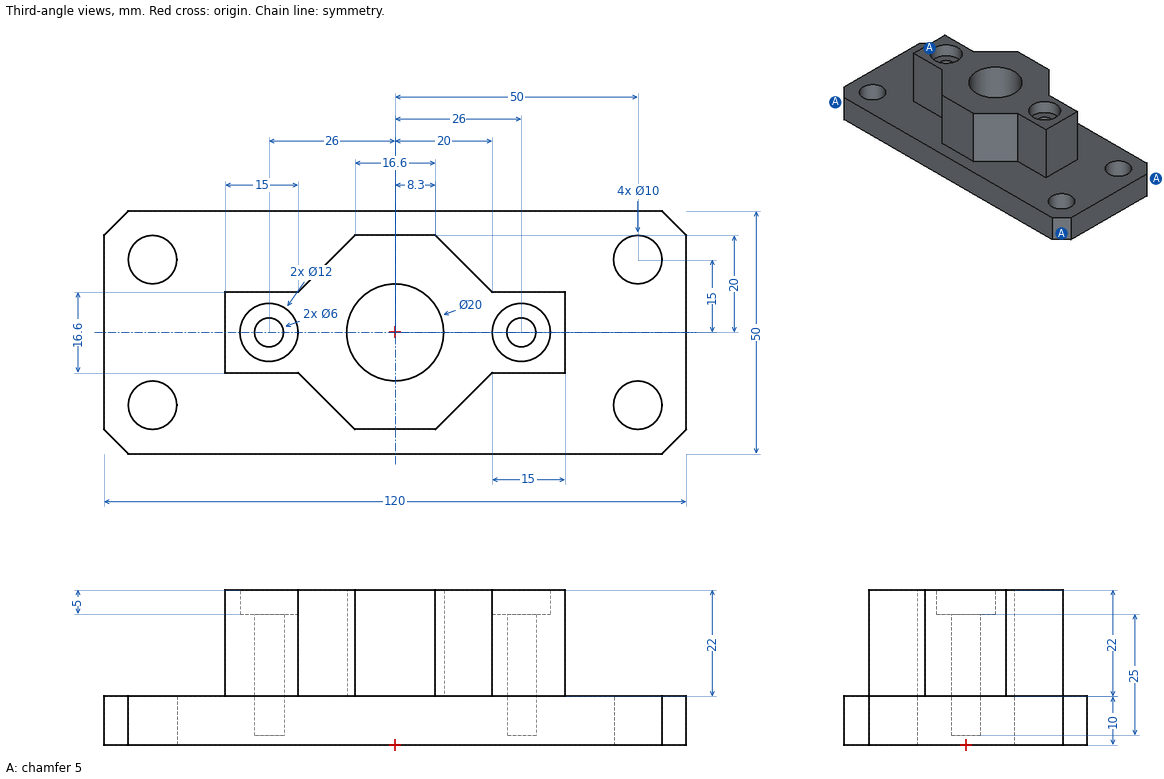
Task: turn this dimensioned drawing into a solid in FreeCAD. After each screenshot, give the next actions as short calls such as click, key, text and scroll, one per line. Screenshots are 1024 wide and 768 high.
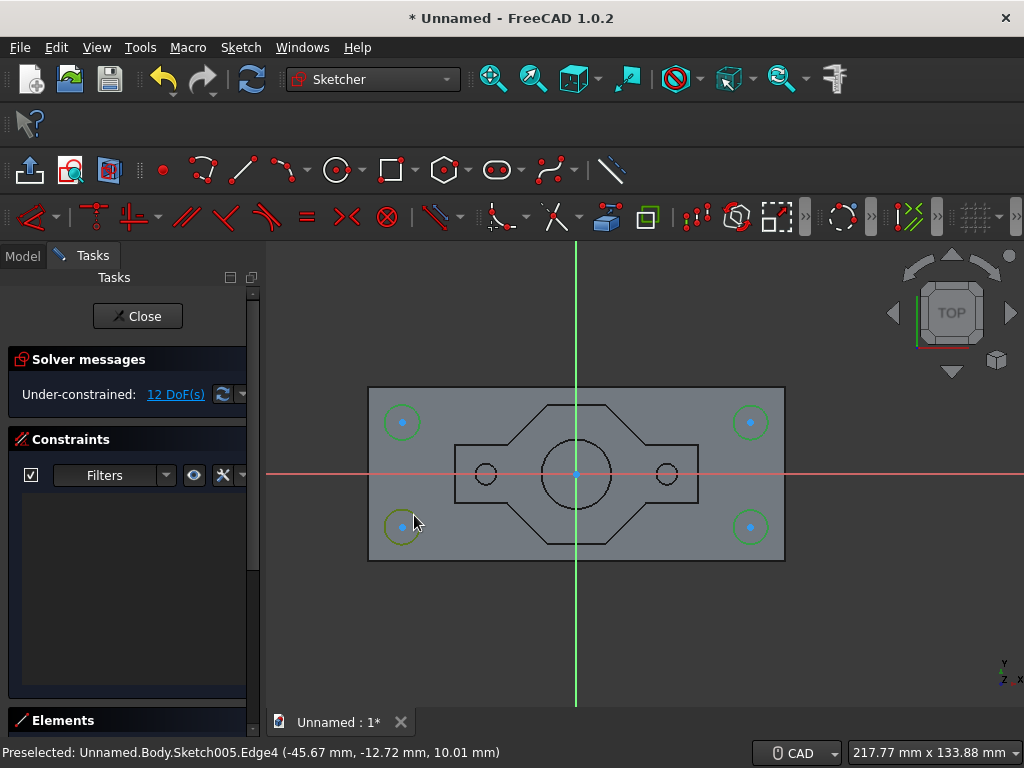
key(e)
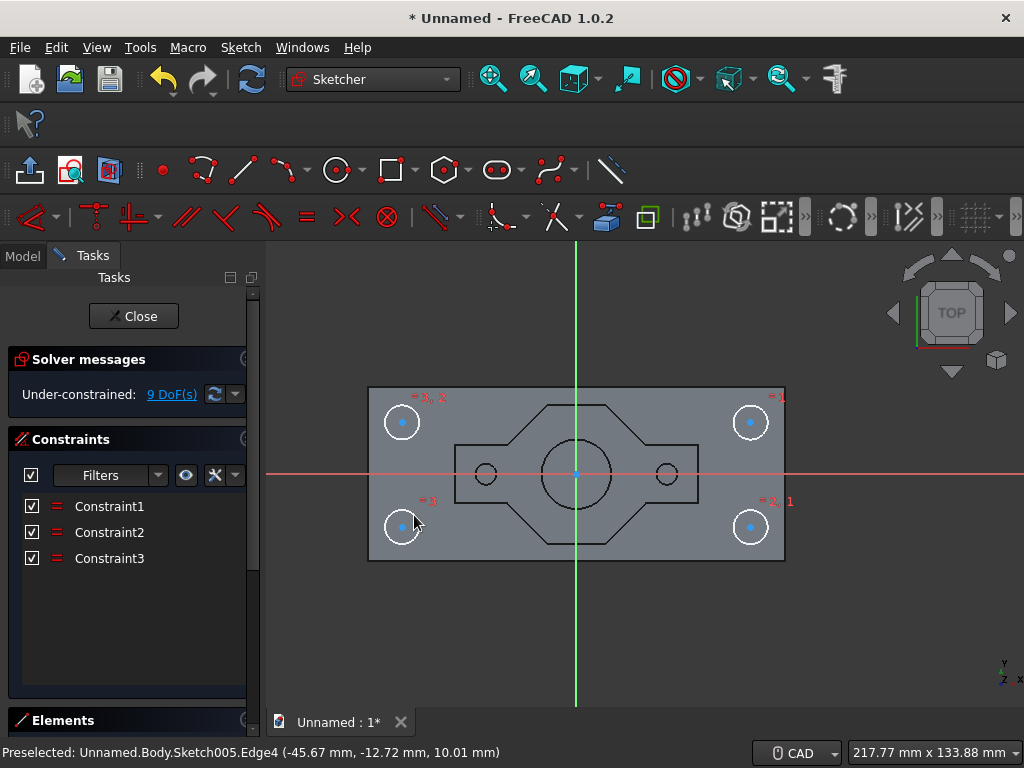
click(751, 423)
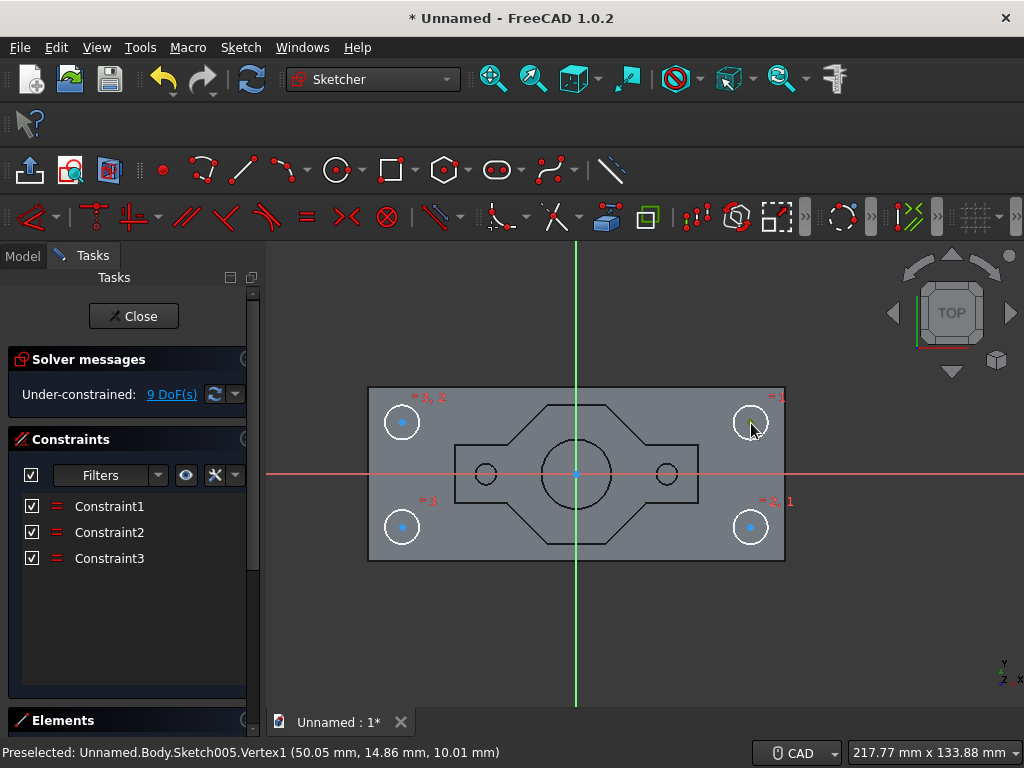
click(751, 527)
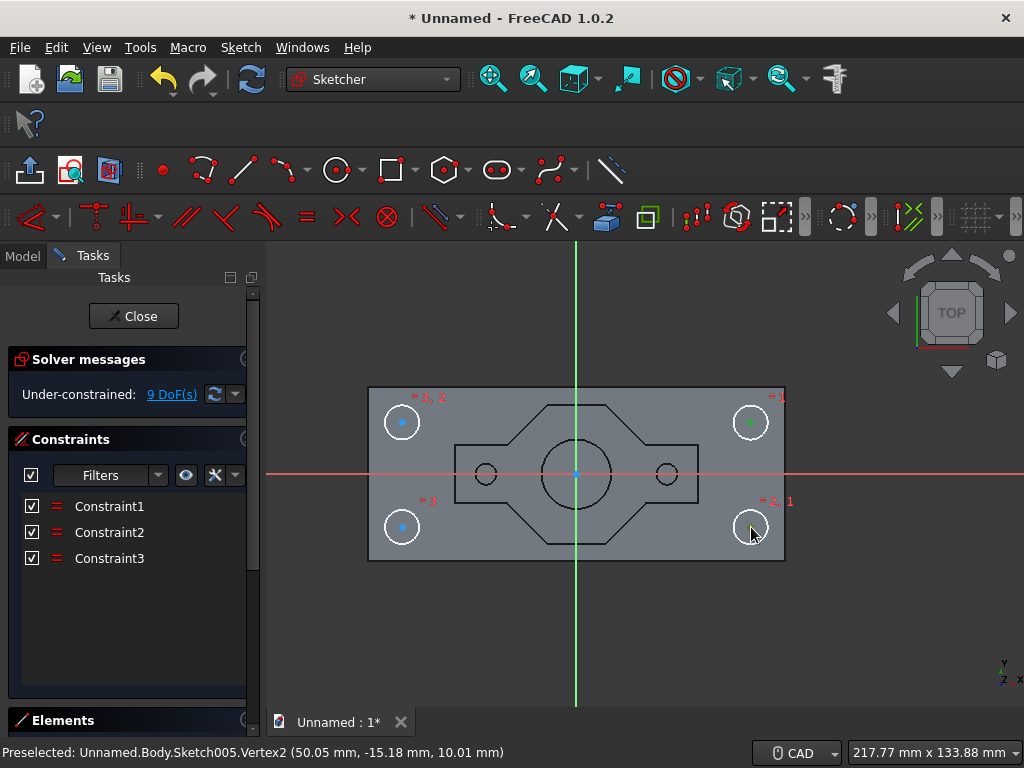
click(334, 474)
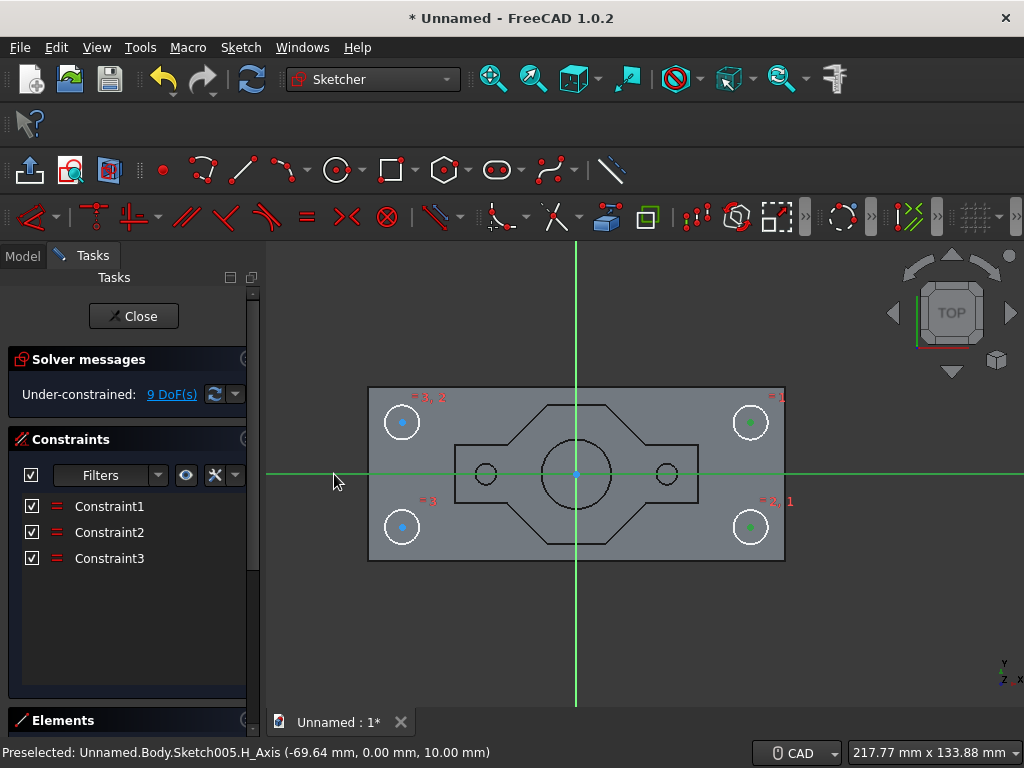
click(348, 218)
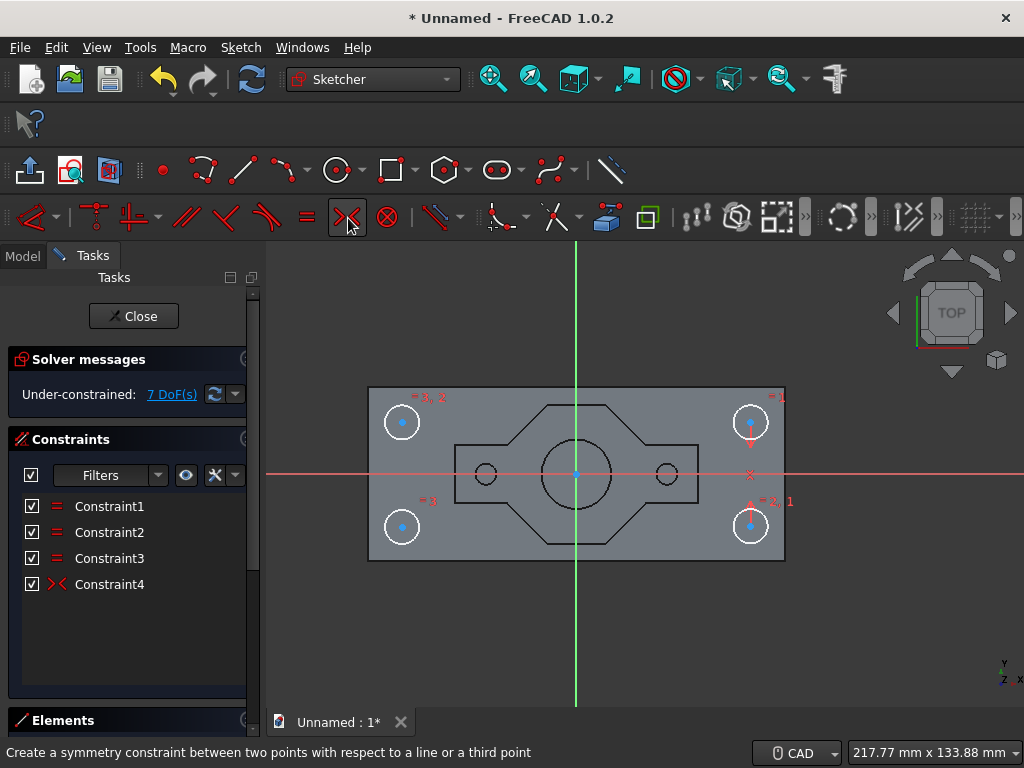
click(751, 422)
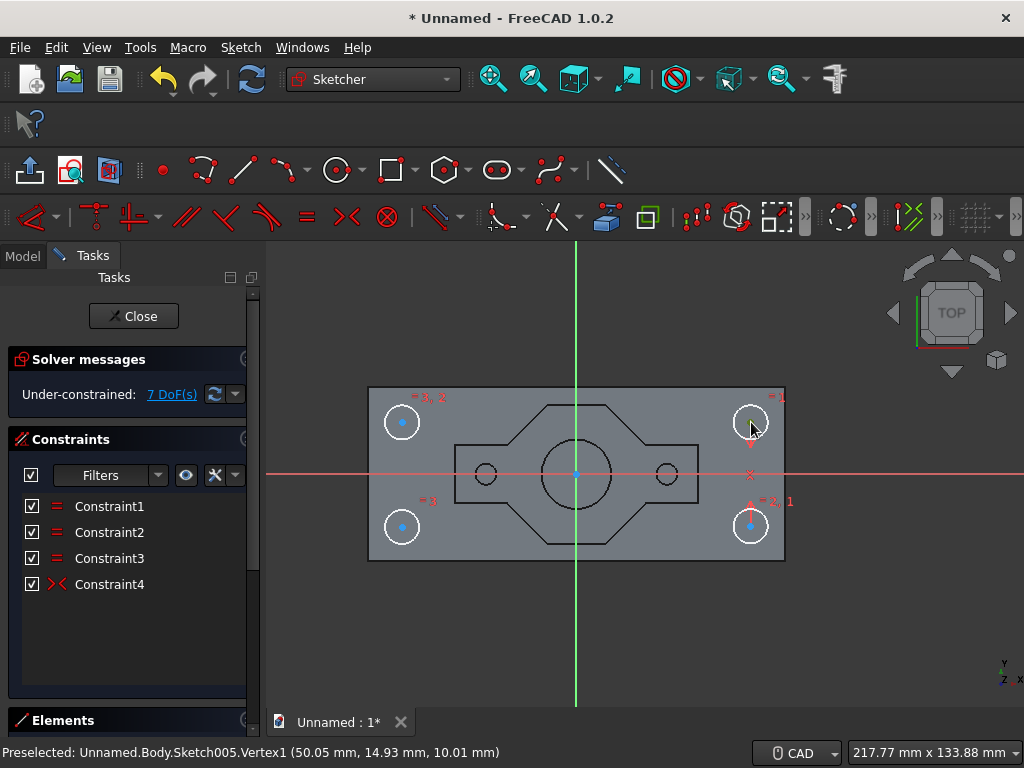
click(402, 422)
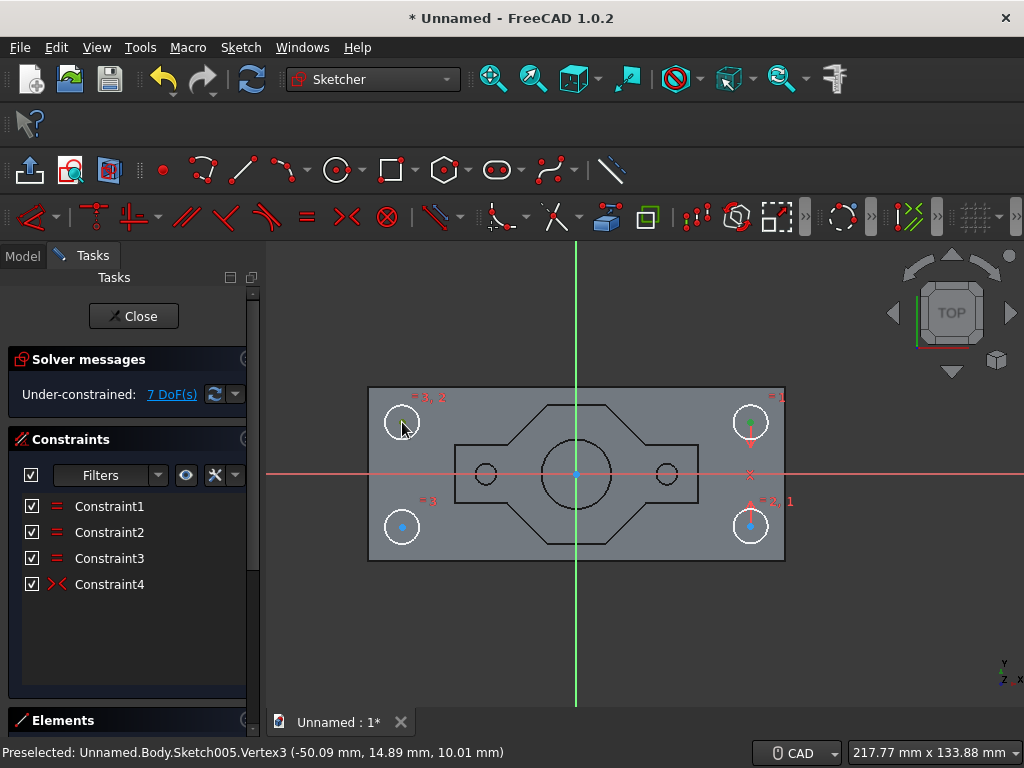
click(576, 650)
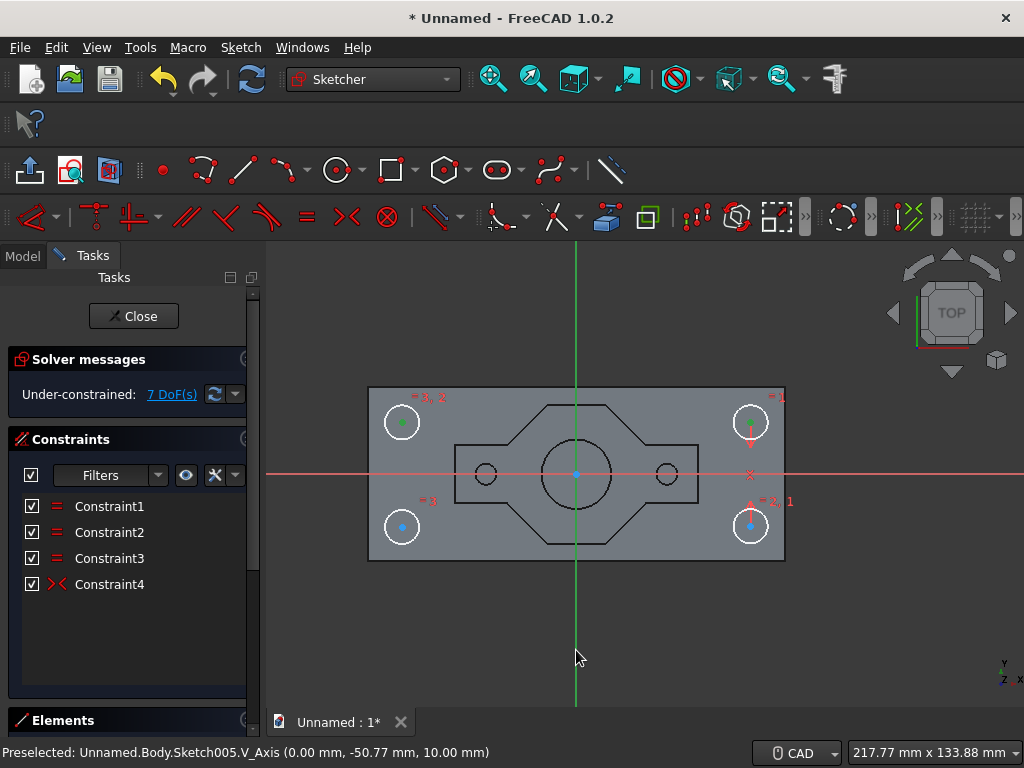
key(s)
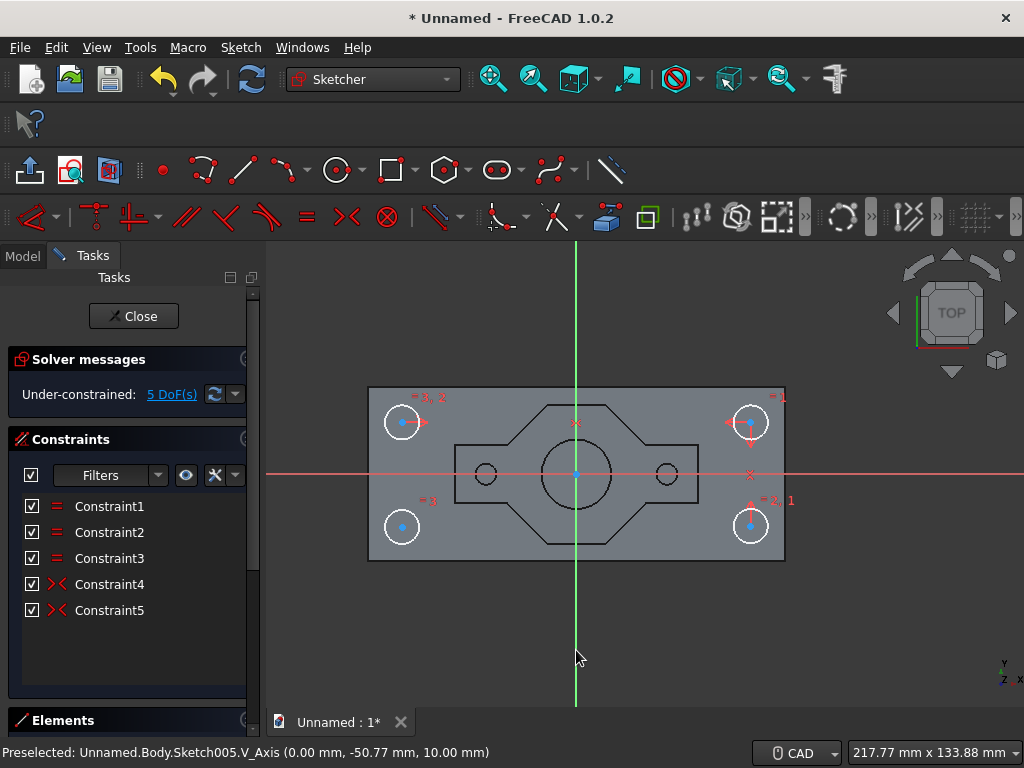
click(751, 526)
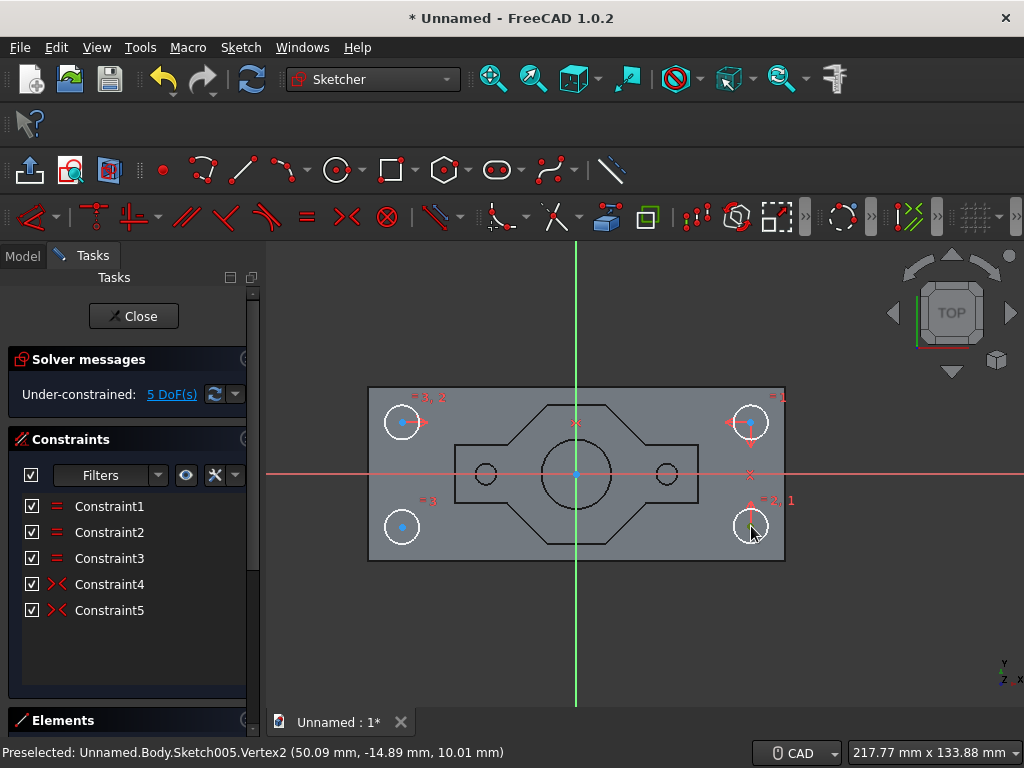
click(402, 527)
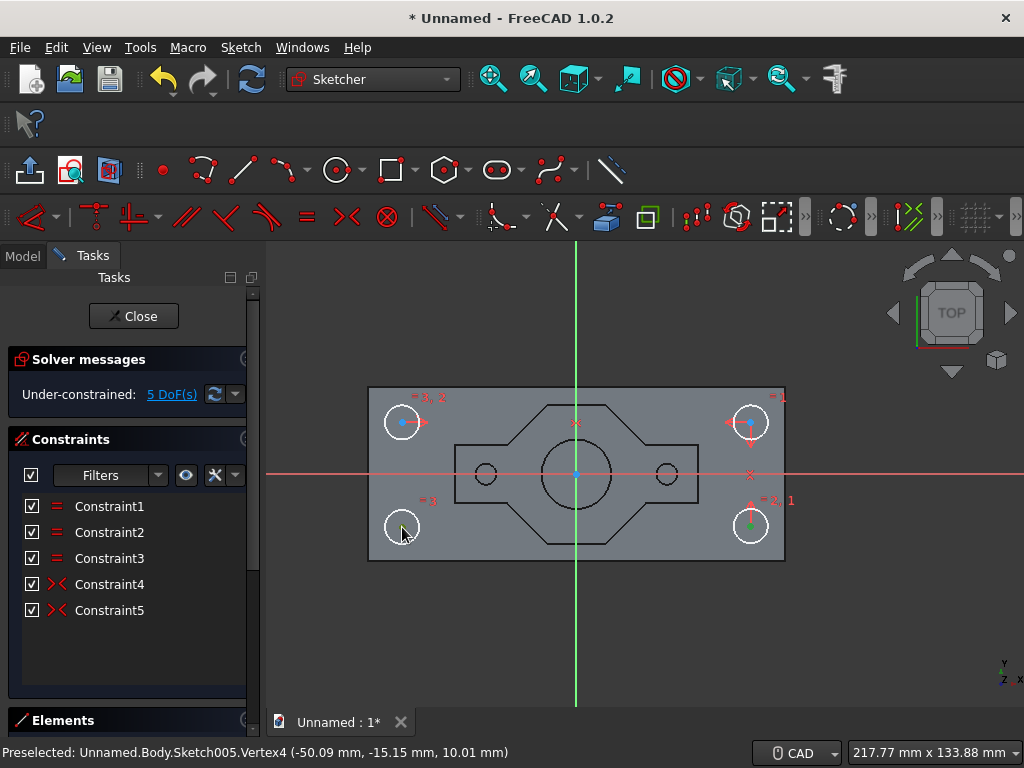
click(576, 650)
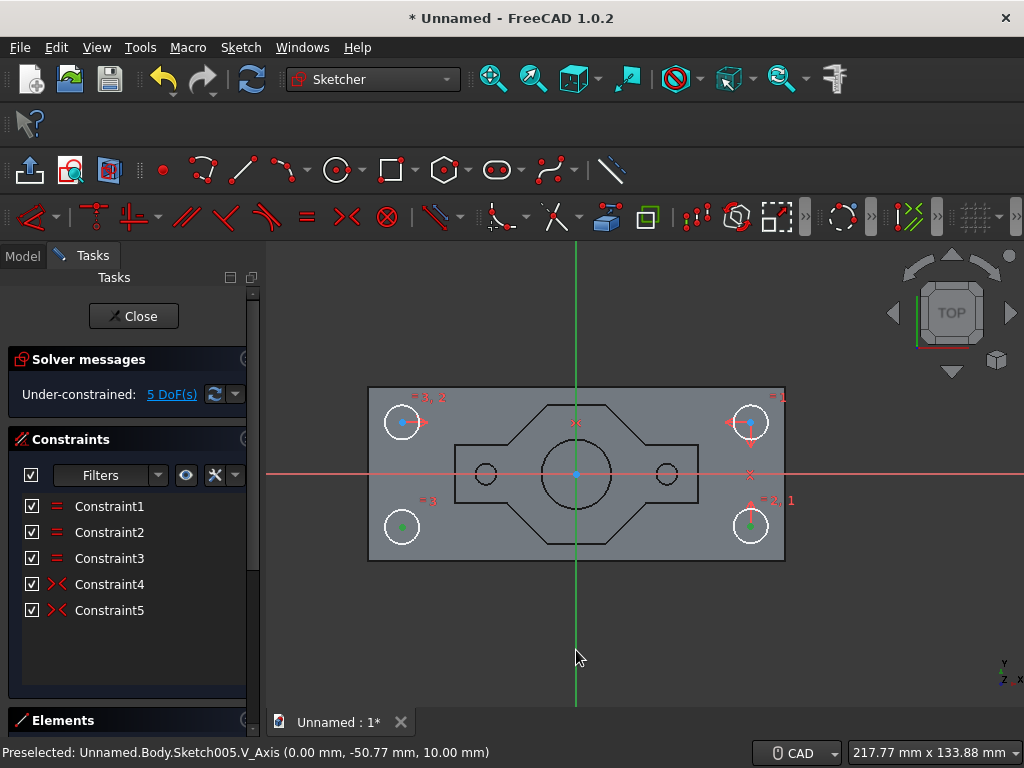
click(348, 218)